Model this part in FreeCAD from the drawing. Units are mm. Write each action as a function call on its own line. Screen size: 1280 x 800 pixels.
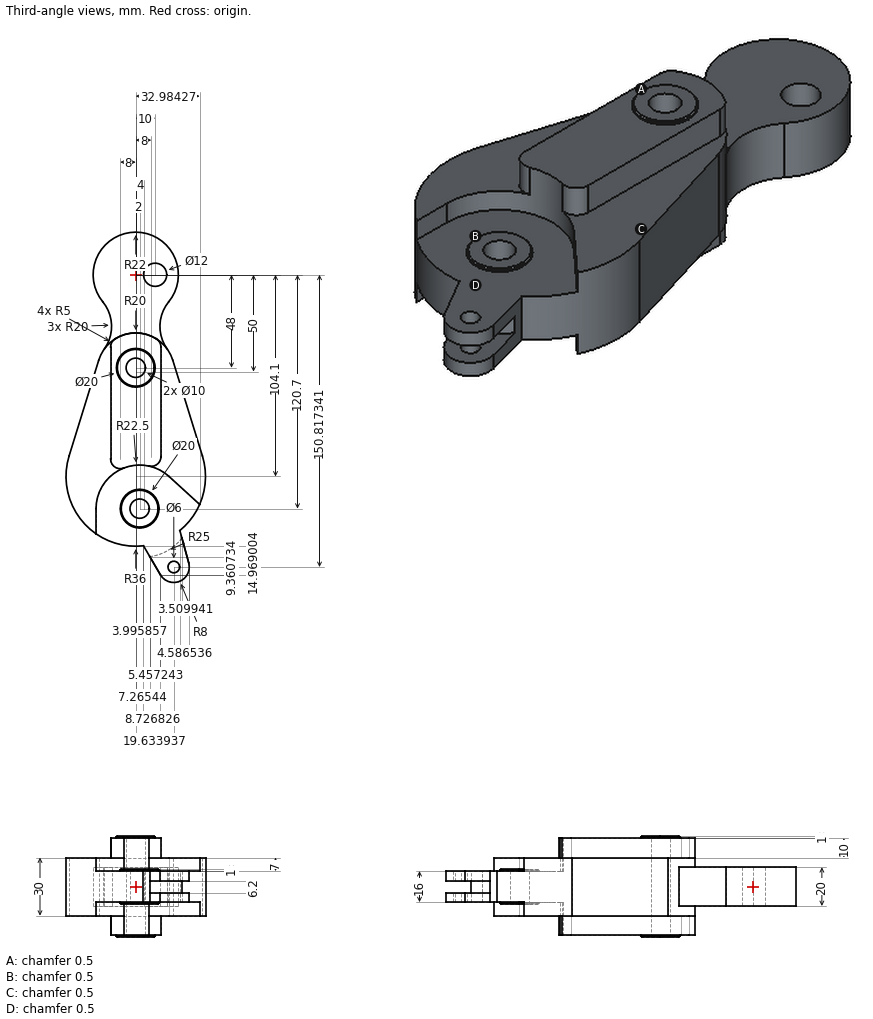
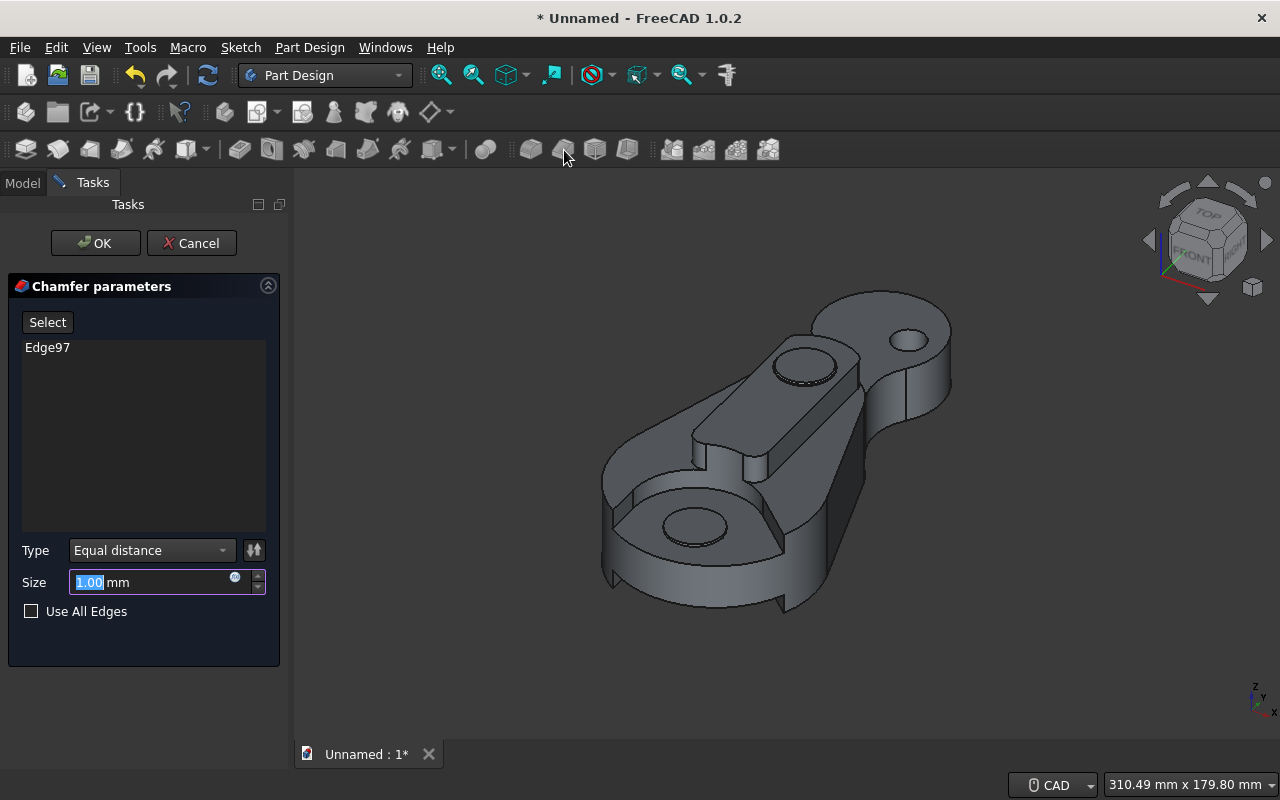
text(0.5)
key(Tab)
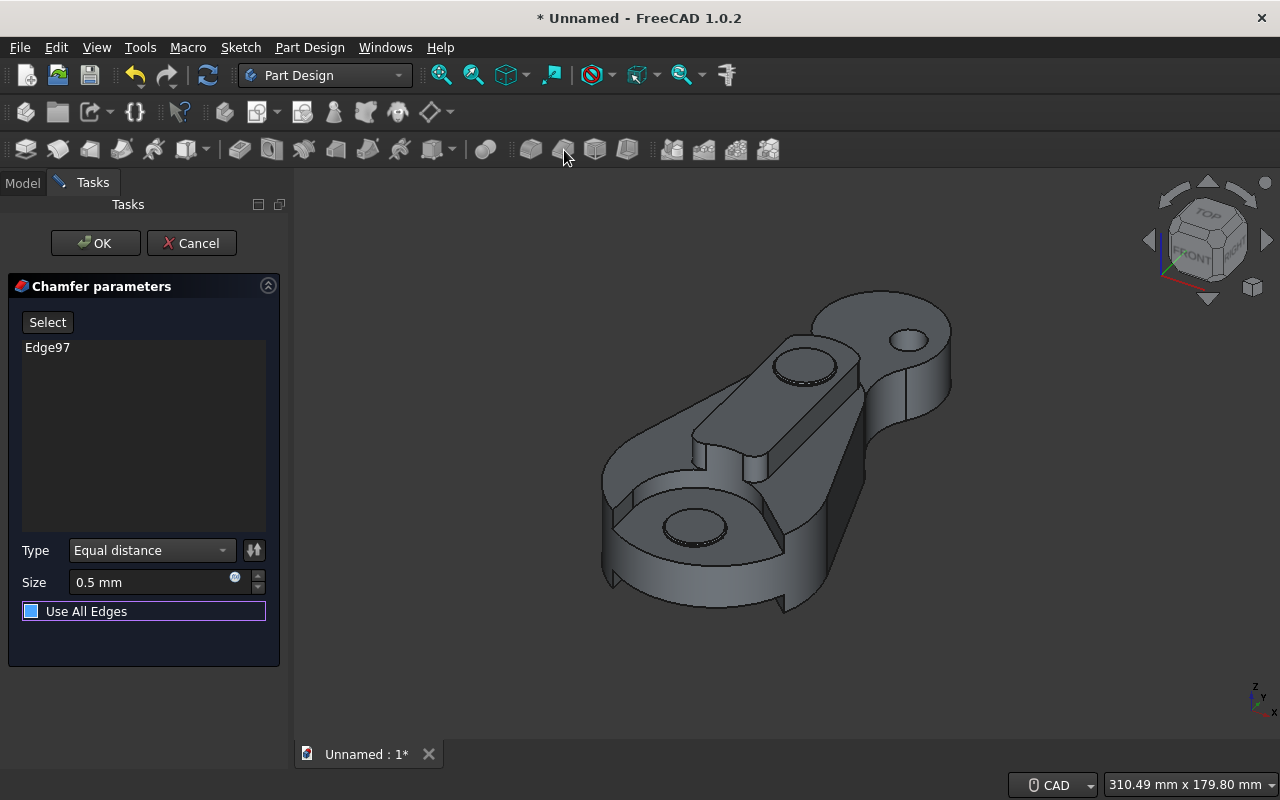
click(96, 243)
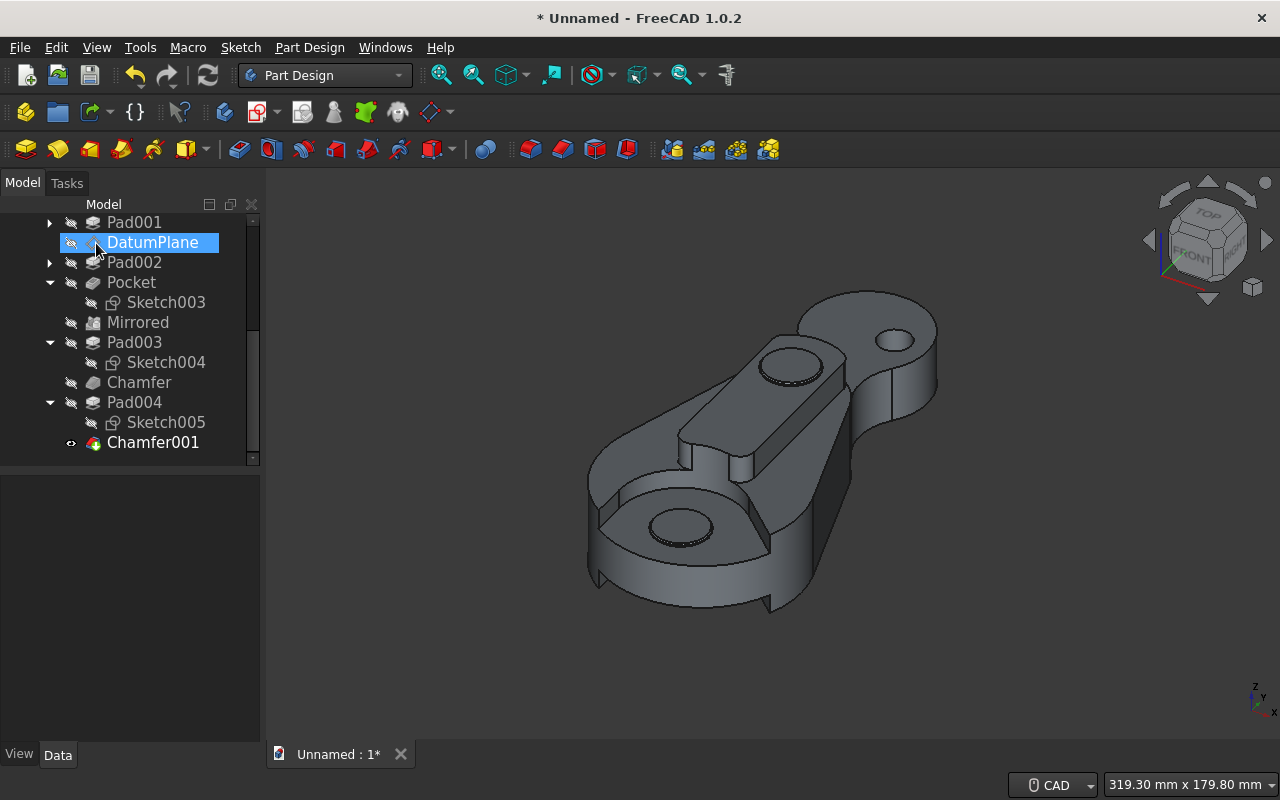
click(116, 343)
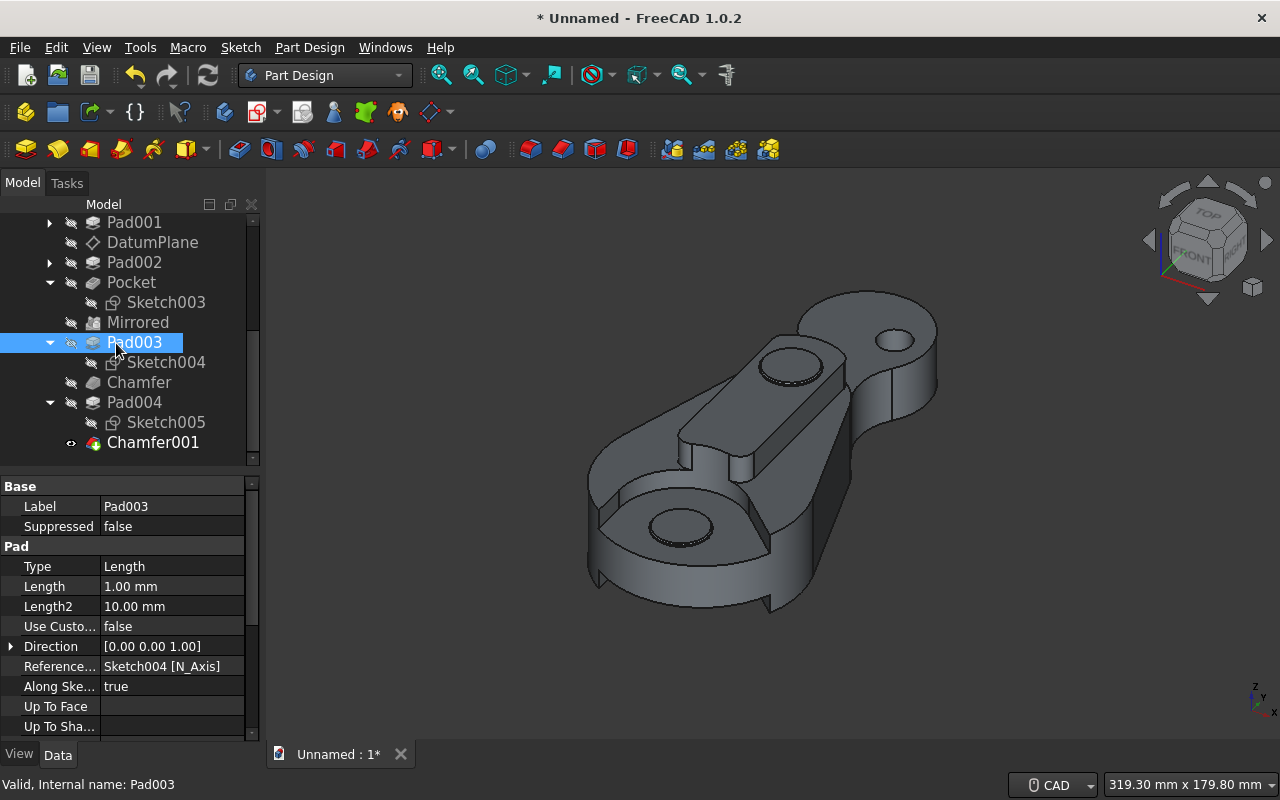
click(116, 403, ctrl)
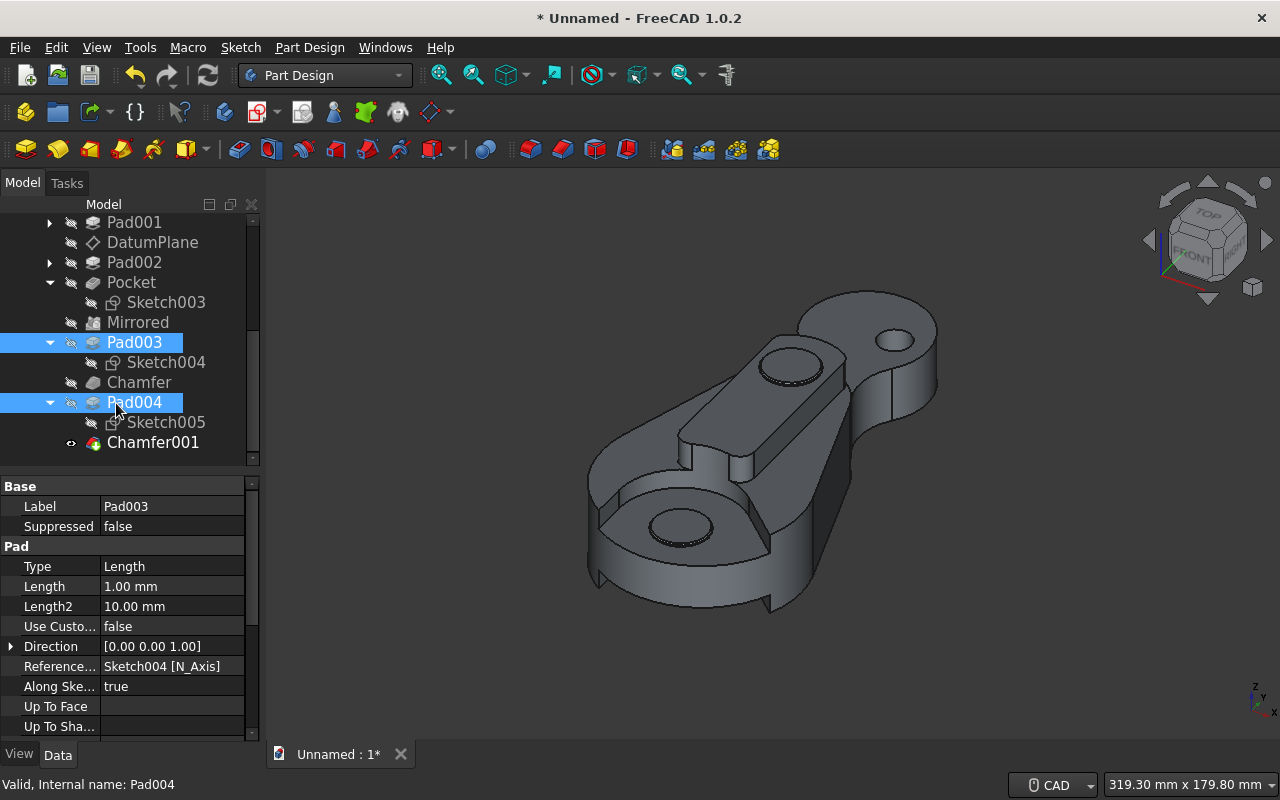
click(672, 150)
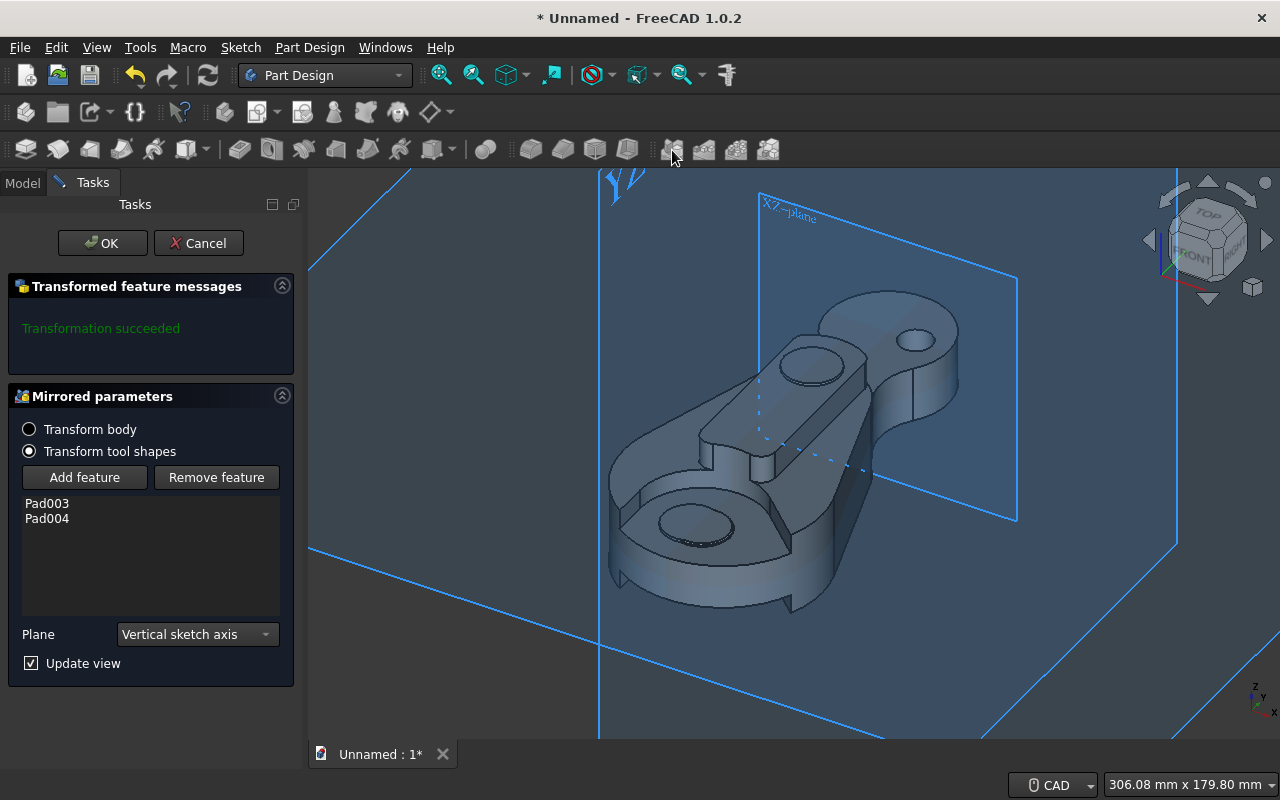
click(198, 634)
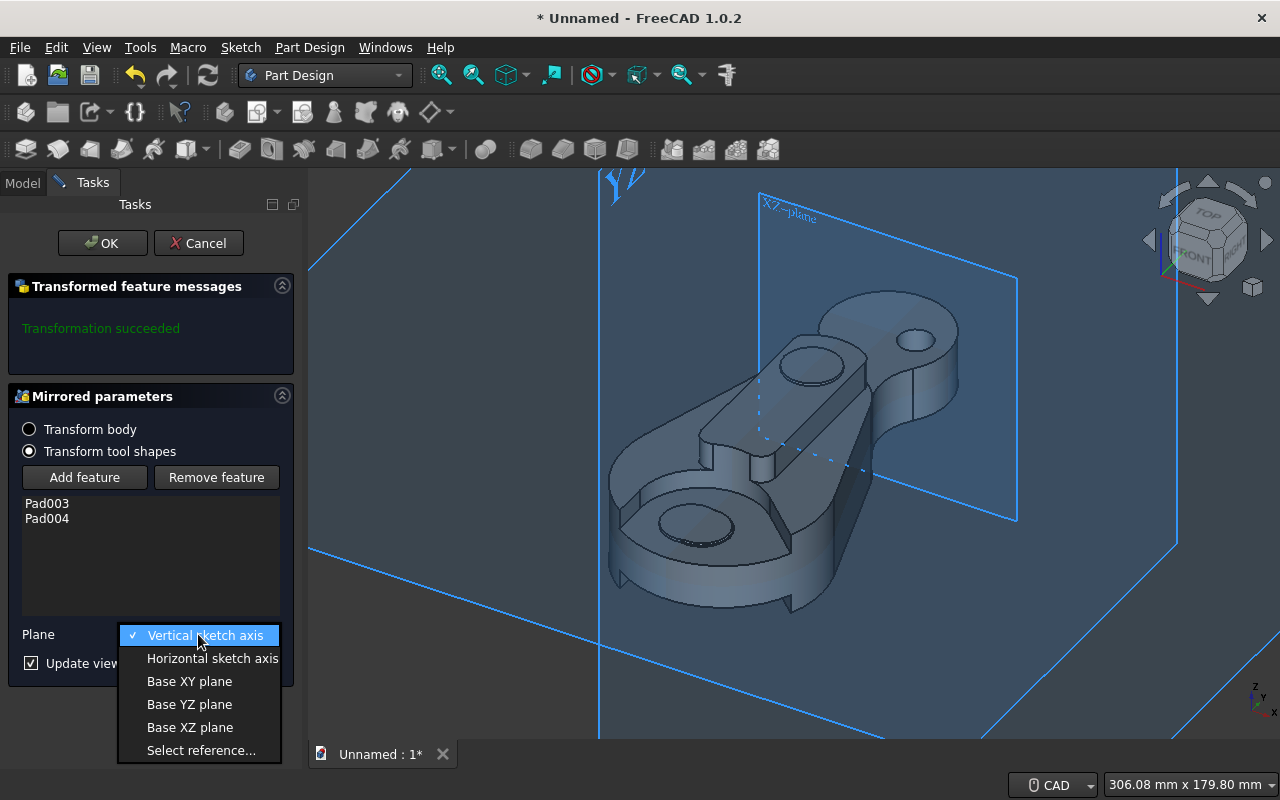
click(198, 682)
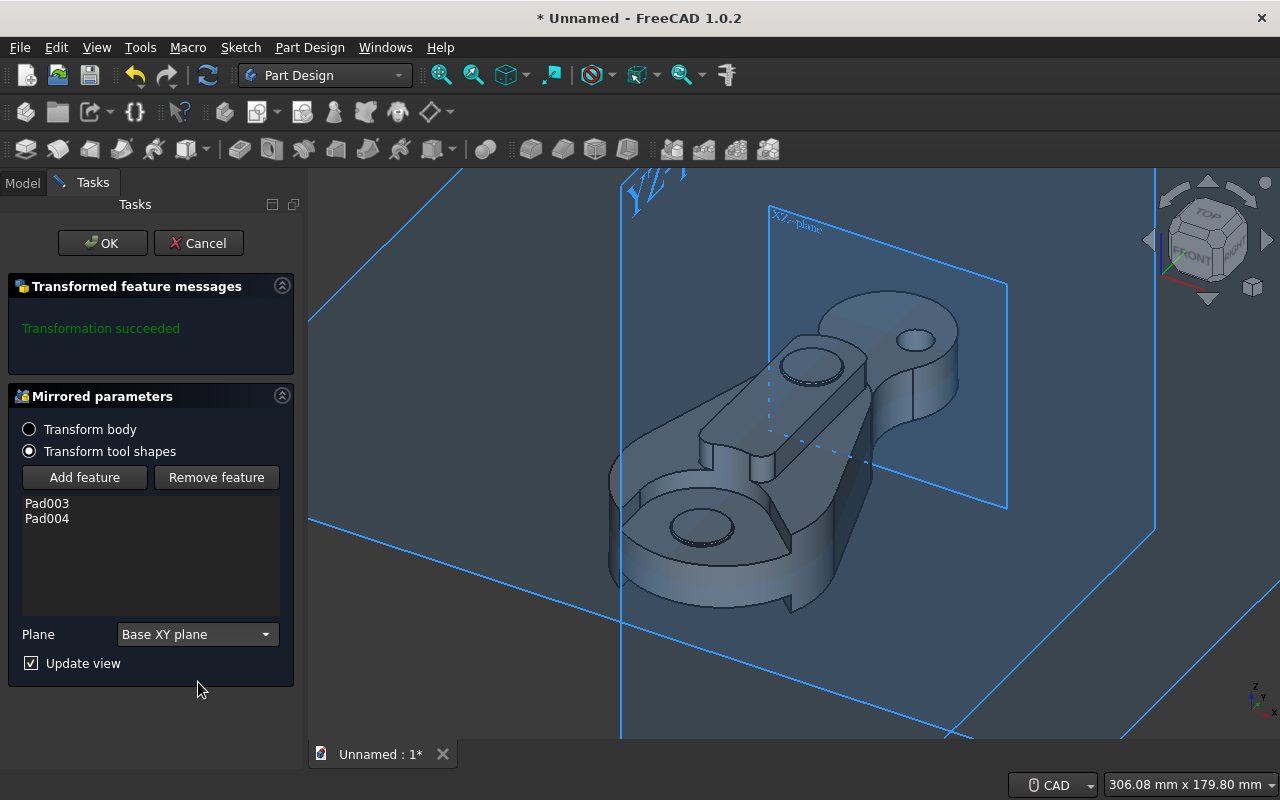
click(103, 243)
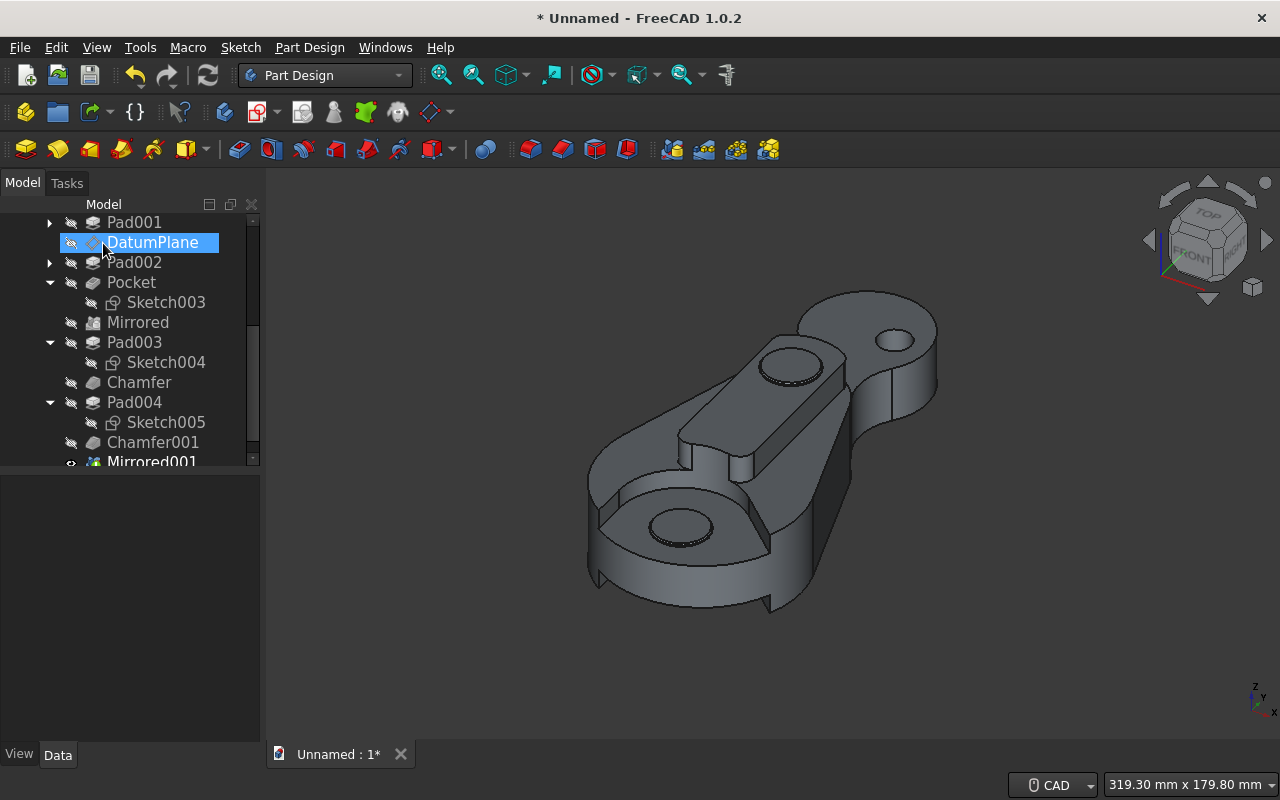
key(0)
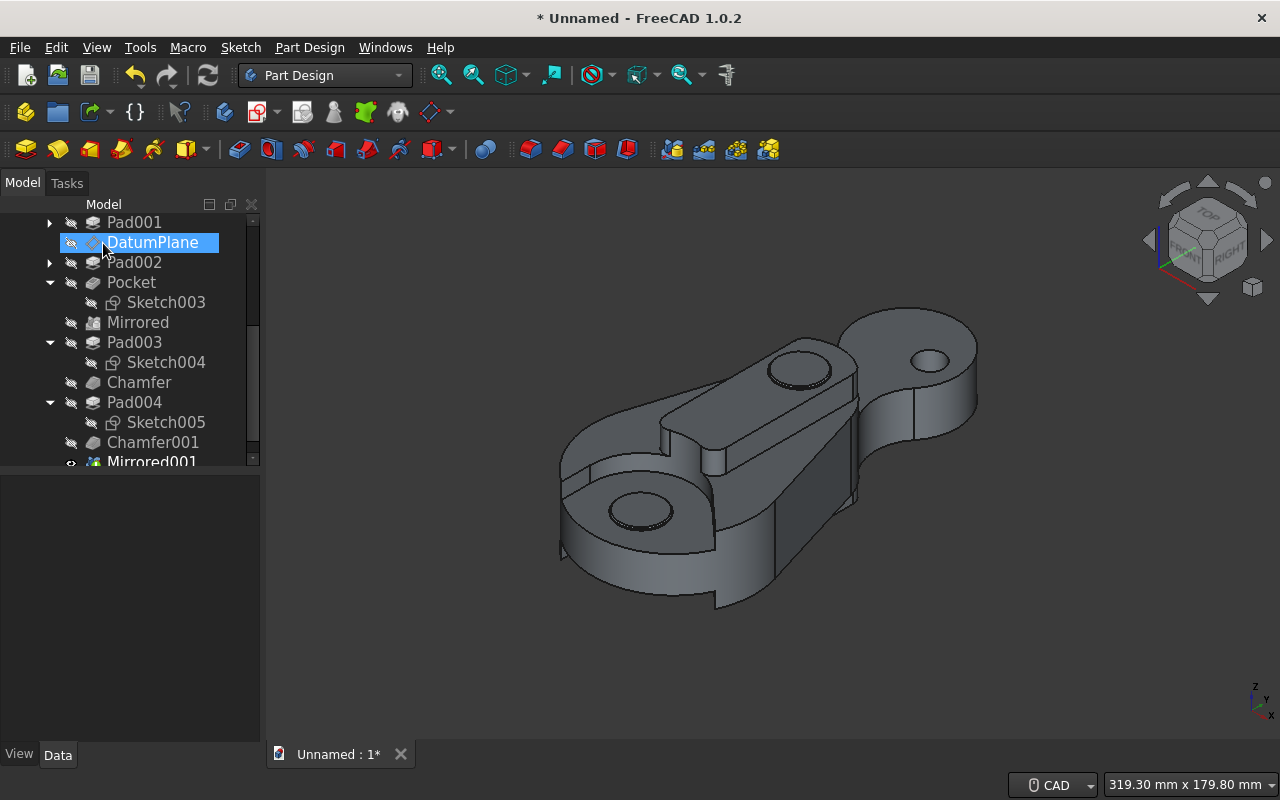
key(2)